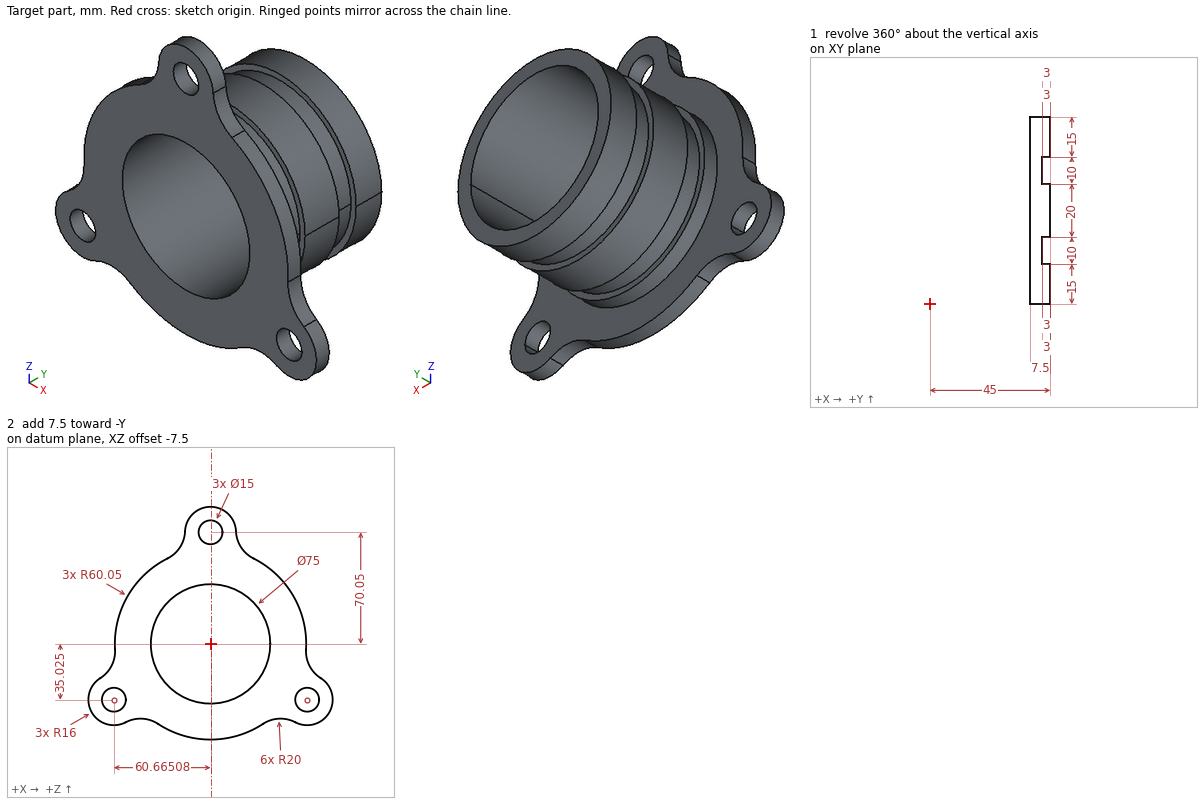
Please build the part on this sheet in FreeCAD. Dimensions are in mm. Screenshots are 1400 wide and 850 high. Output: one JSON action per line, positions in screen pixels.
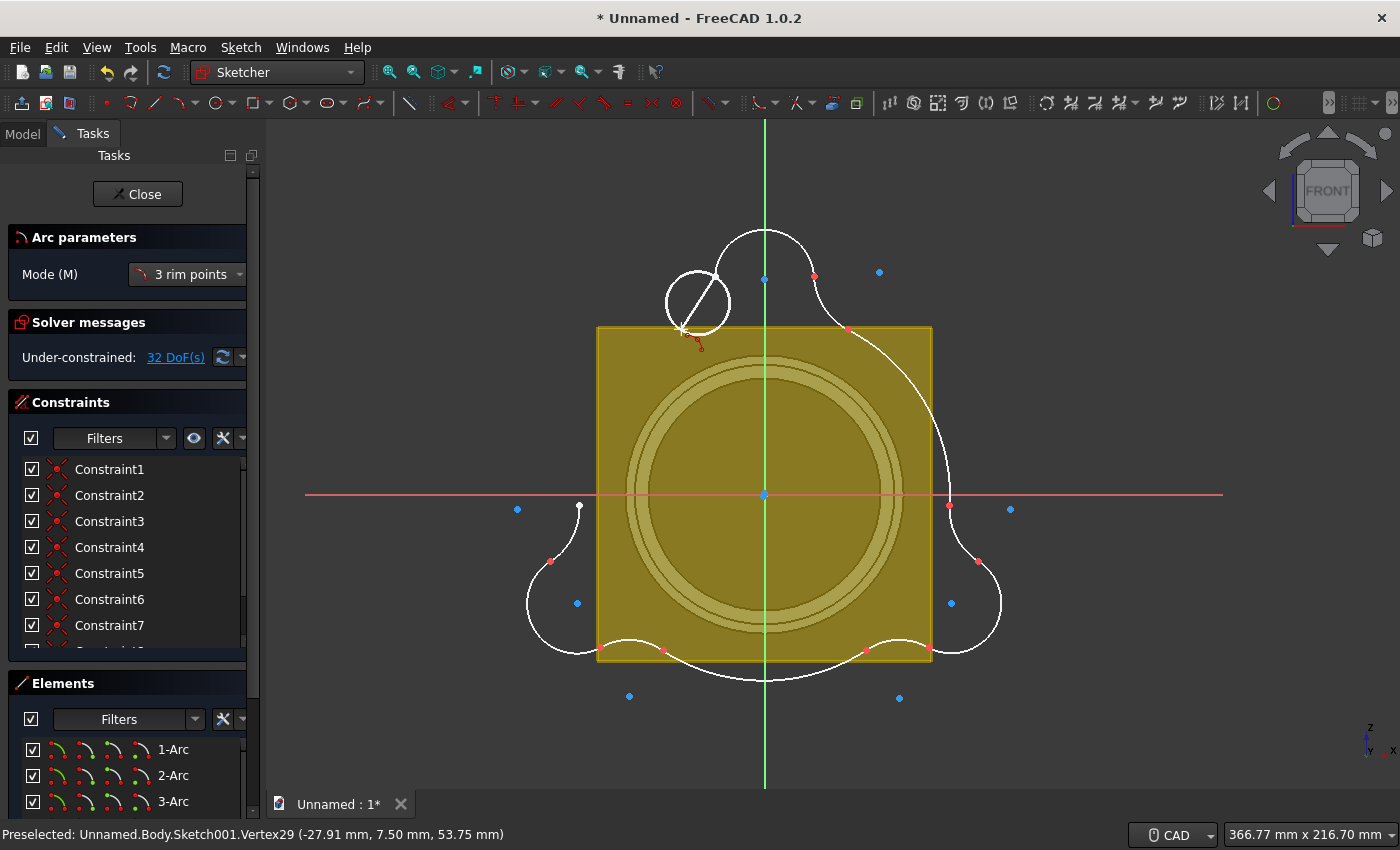
{"action": "scroll", "coordinate": [705, 307], "scroll_direction": "up", "scroll_amount": 4}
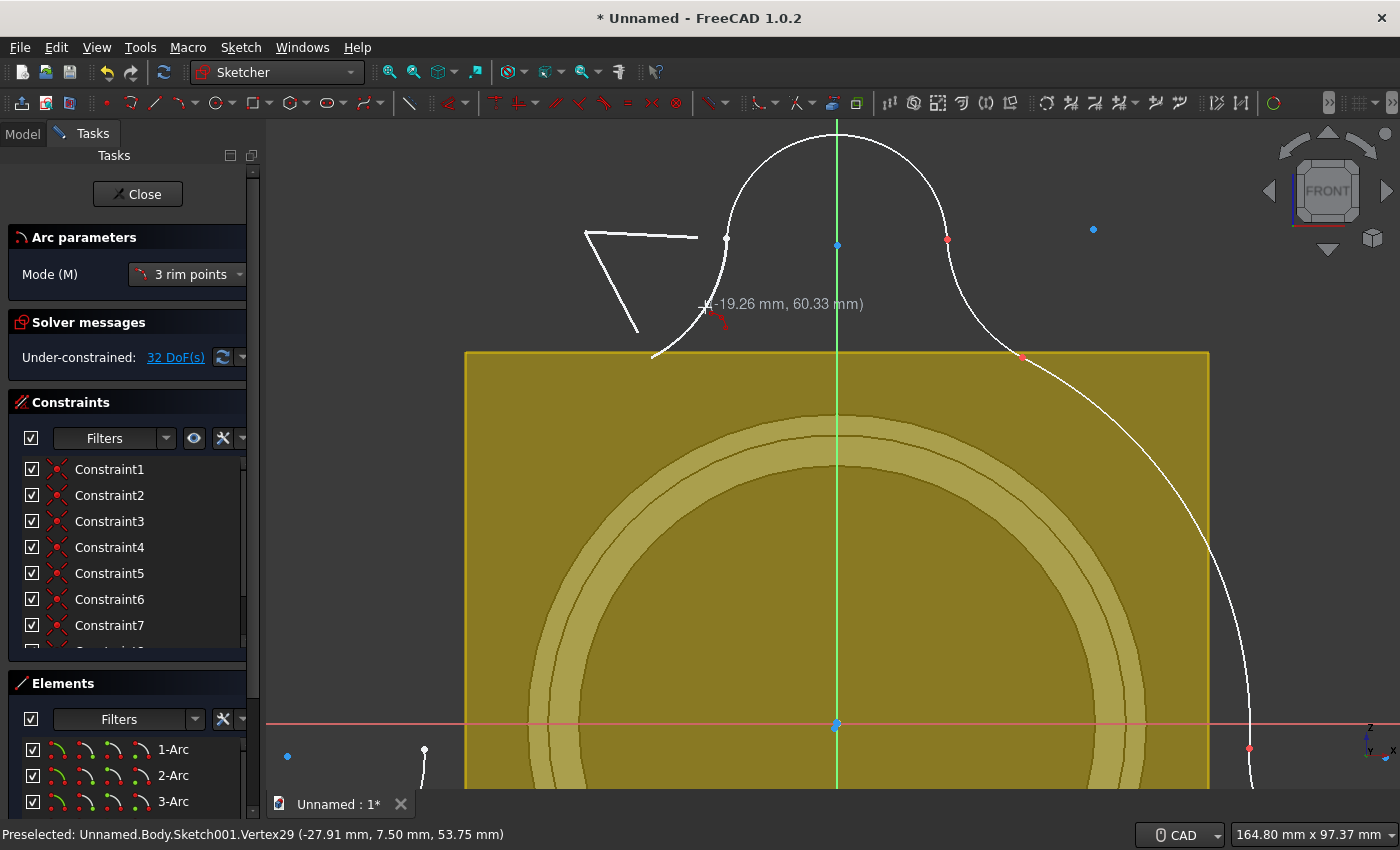
{"action": "left_click", "coordinate": [705, 306]}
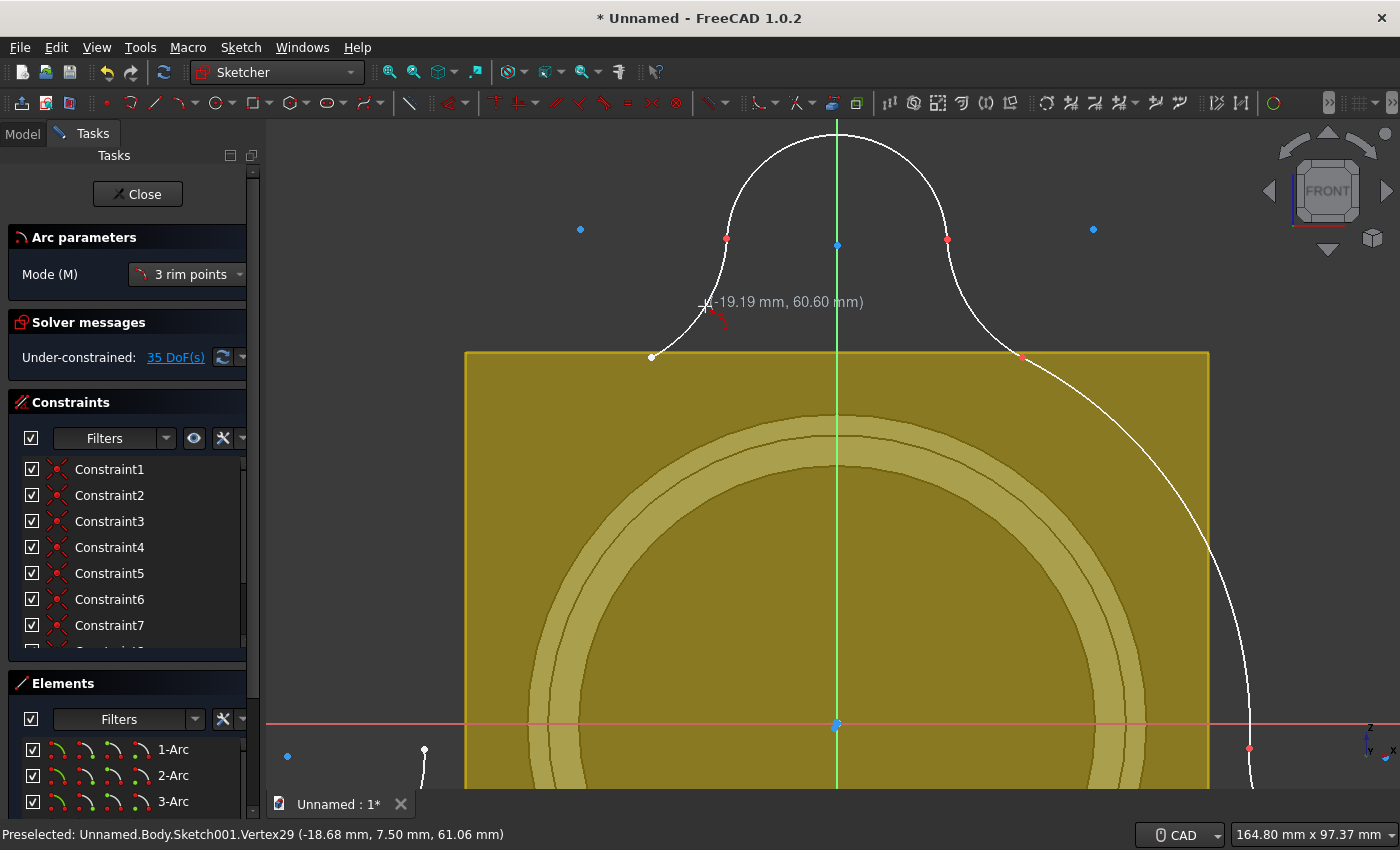
{"action": "left_click", "coordinate": [651, 358]}
{"action": "left_click", "coordinate": [424, 749]}
{"action": "left_click", "coordinate": [479, 517]}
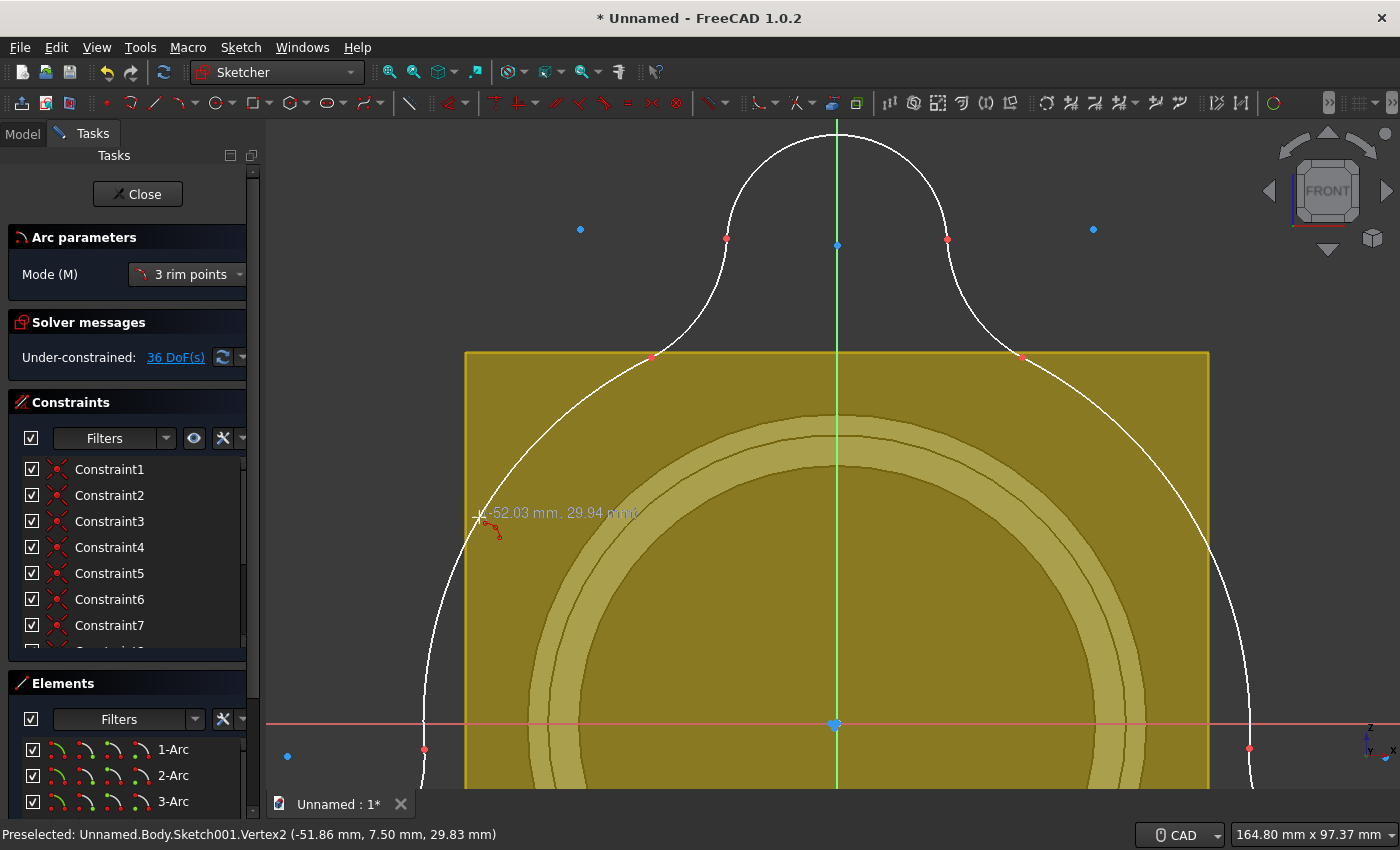
{"action": "left_click", "coordinate": [216, 104]}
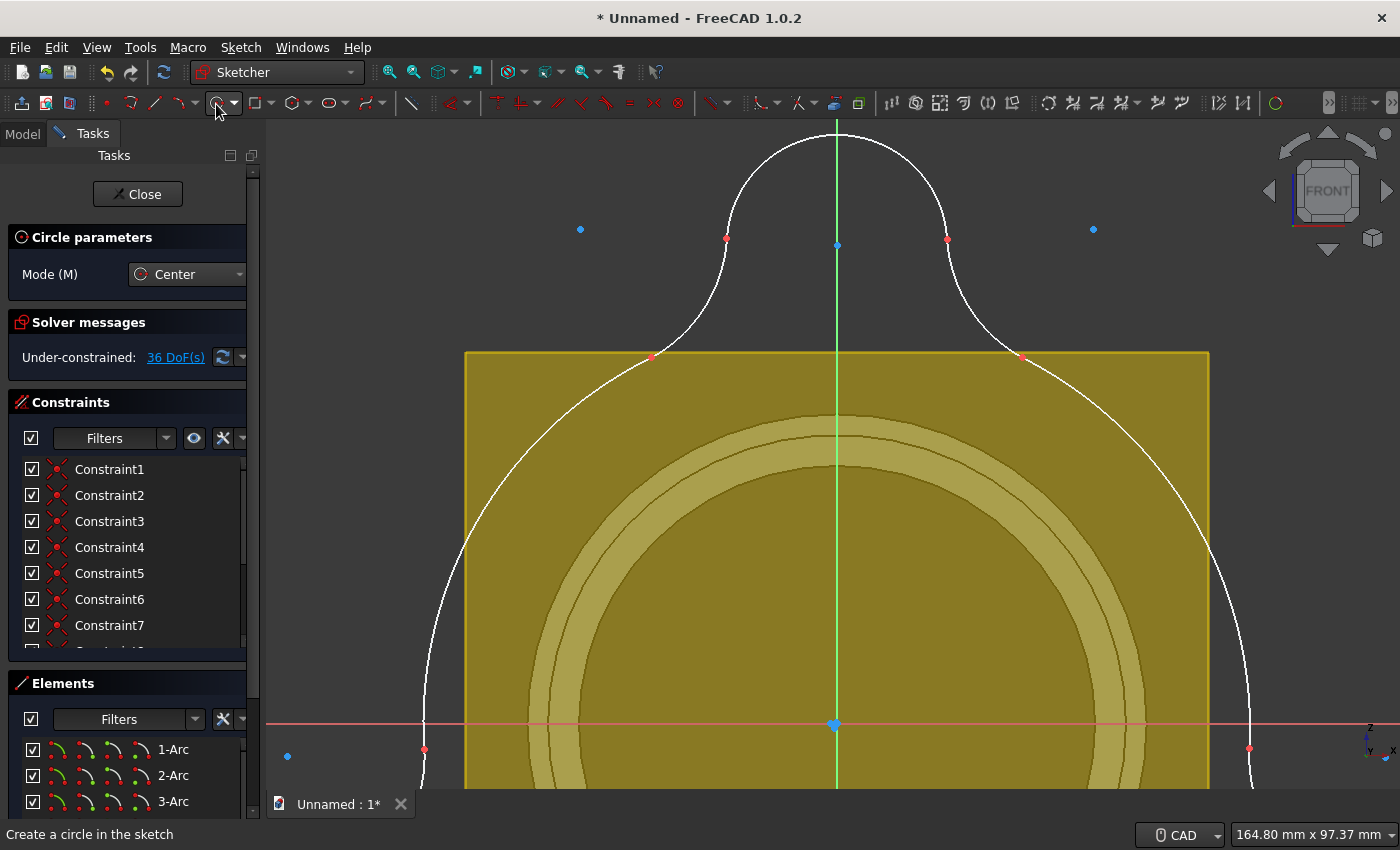
{"action": "scroll", "coordinate": [705, 307], "scroll_direction": "down", "scroll_amount": 4}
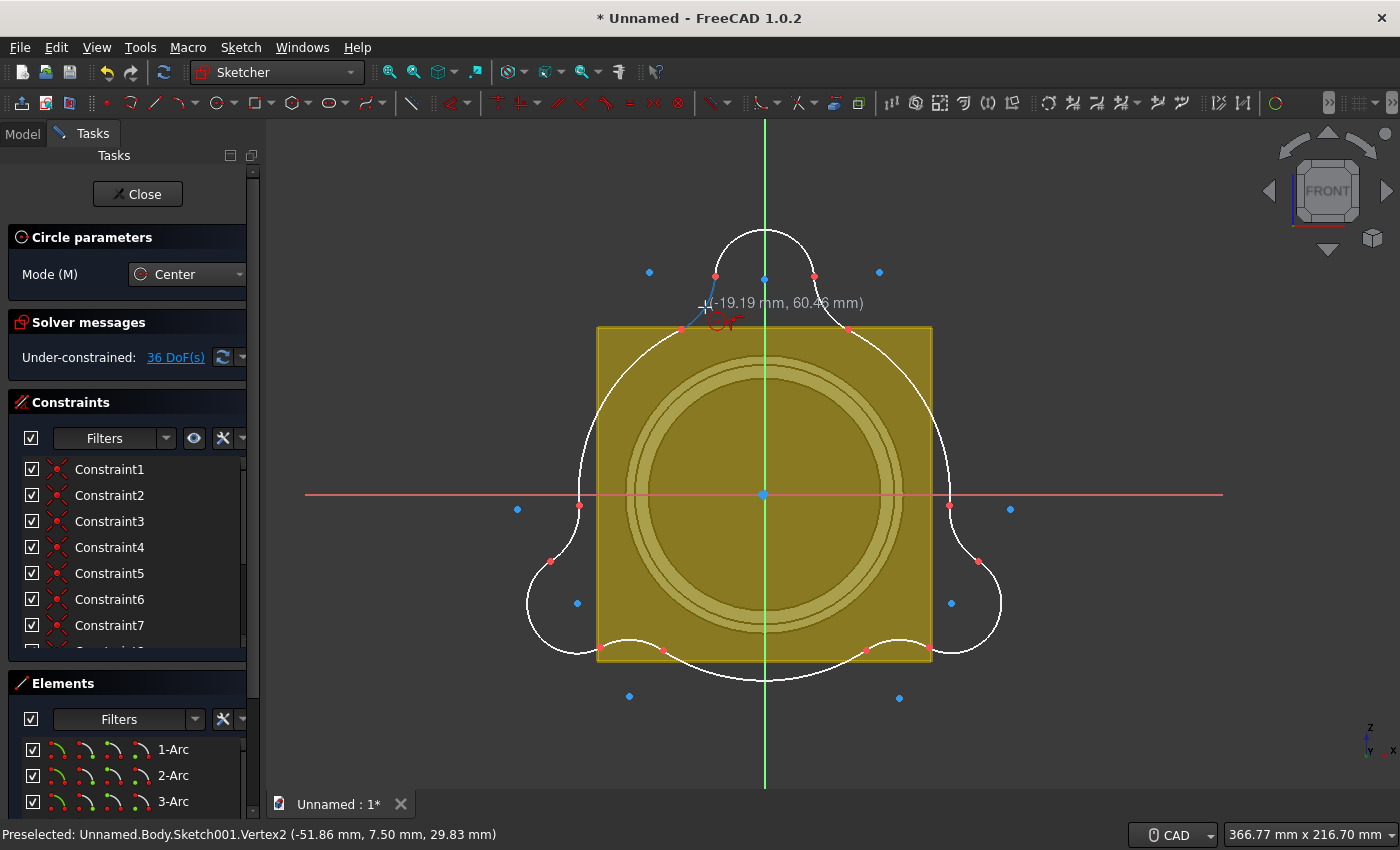
{"action": "left_click", "coordinate": [577, 603]}
{"action": "left_click", "coordinate": [593, 586]}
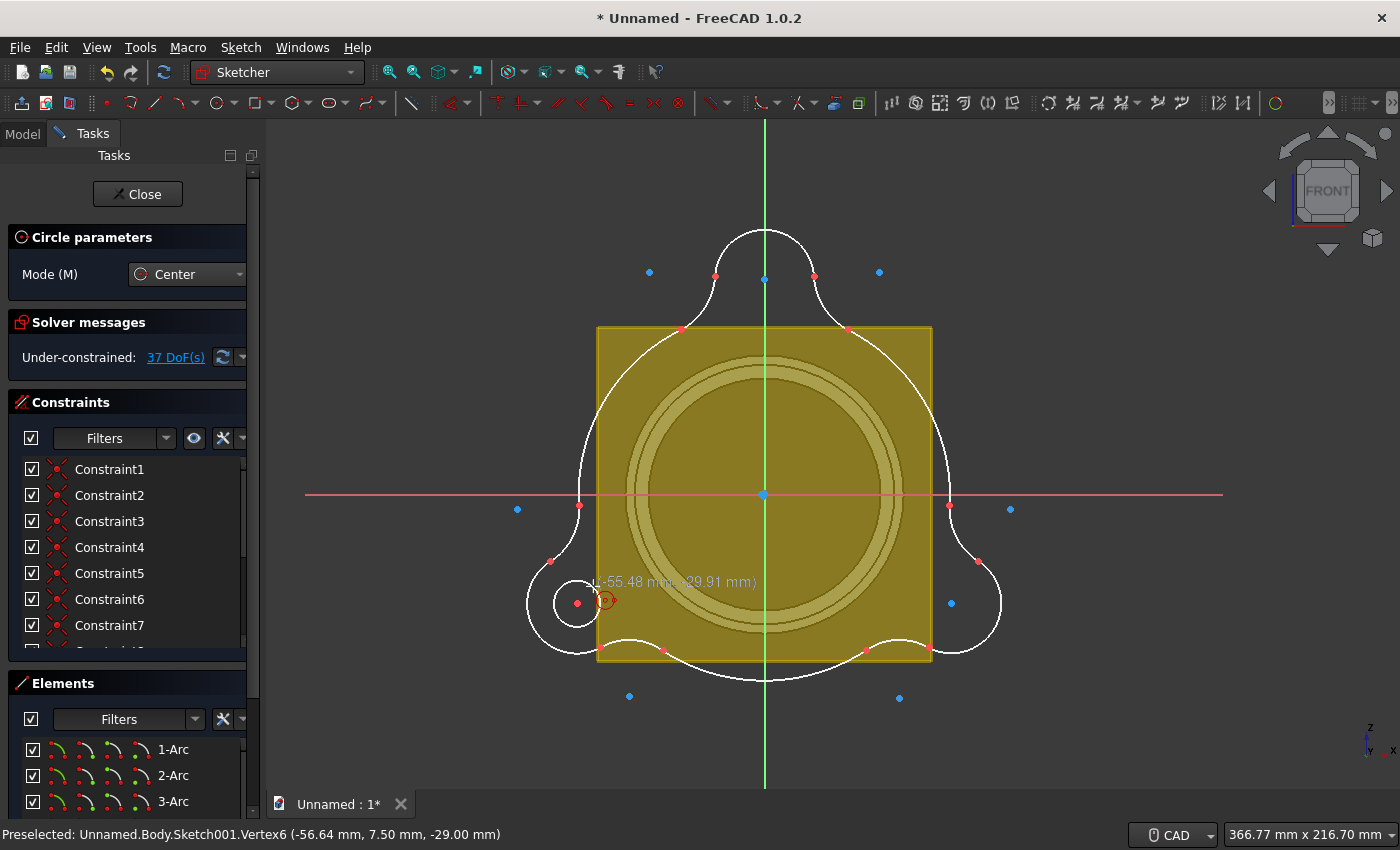
{"action": "left_click", "coordinate": [952, 603]}
{"action": "left_click", "coordinate": [969, 586]}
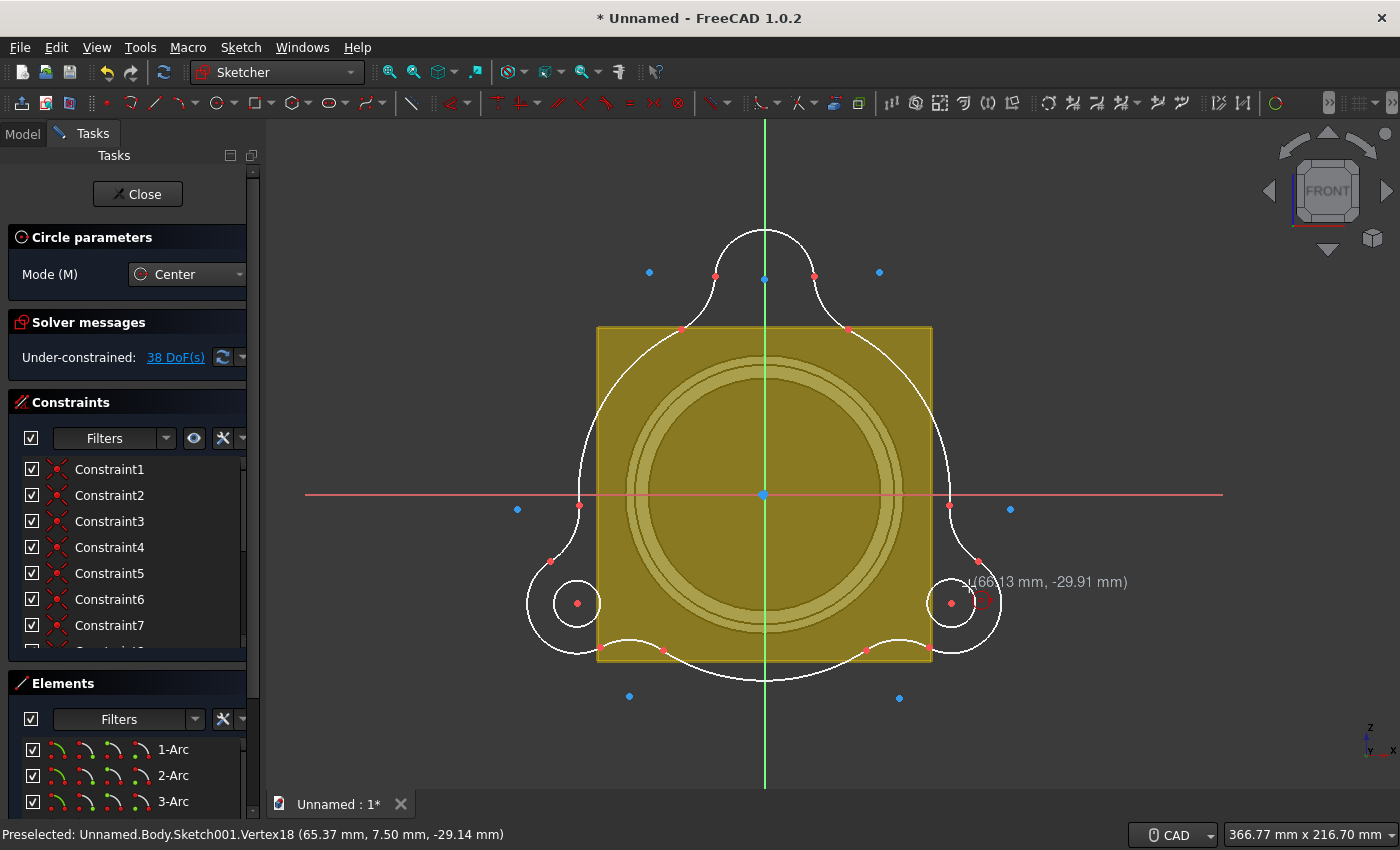
{"action": "left_click", "coordinate": [765, 495]}
{"action": "left_click", "coordinate": [847, 413]}